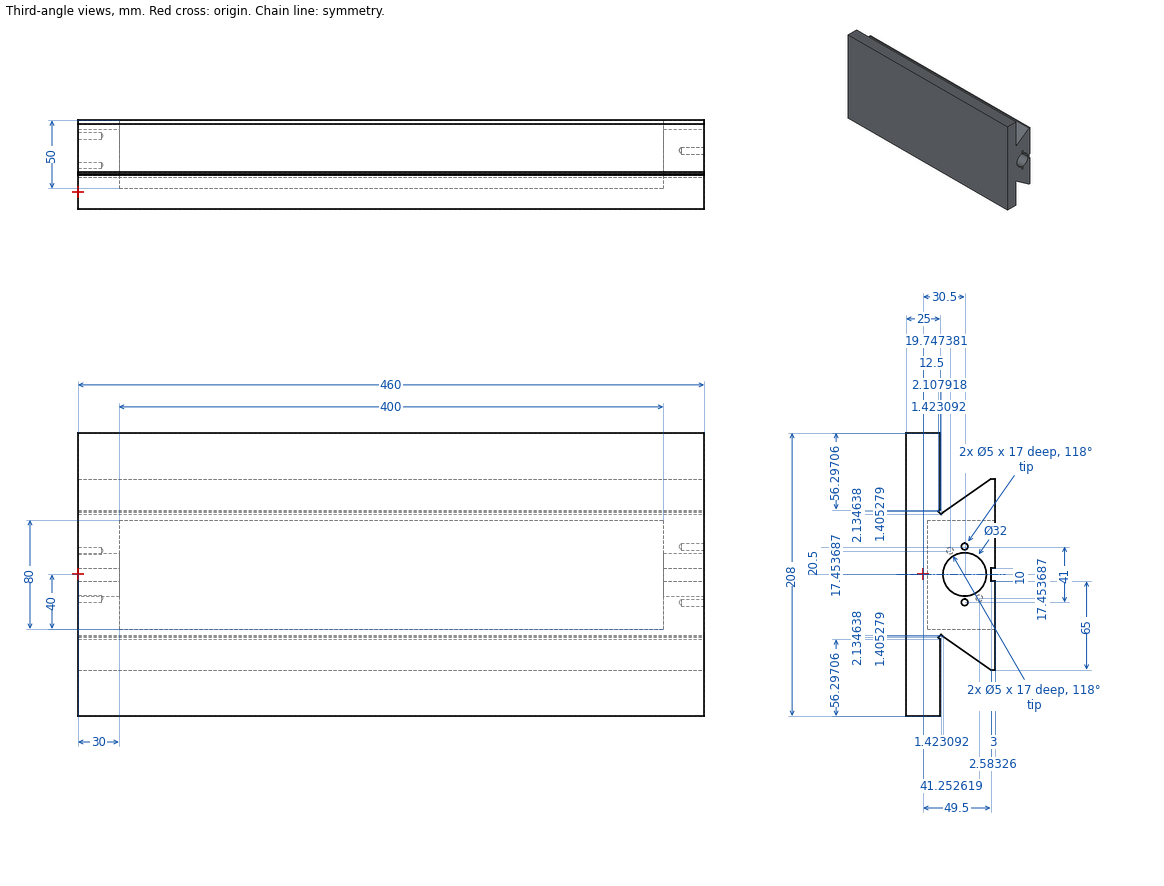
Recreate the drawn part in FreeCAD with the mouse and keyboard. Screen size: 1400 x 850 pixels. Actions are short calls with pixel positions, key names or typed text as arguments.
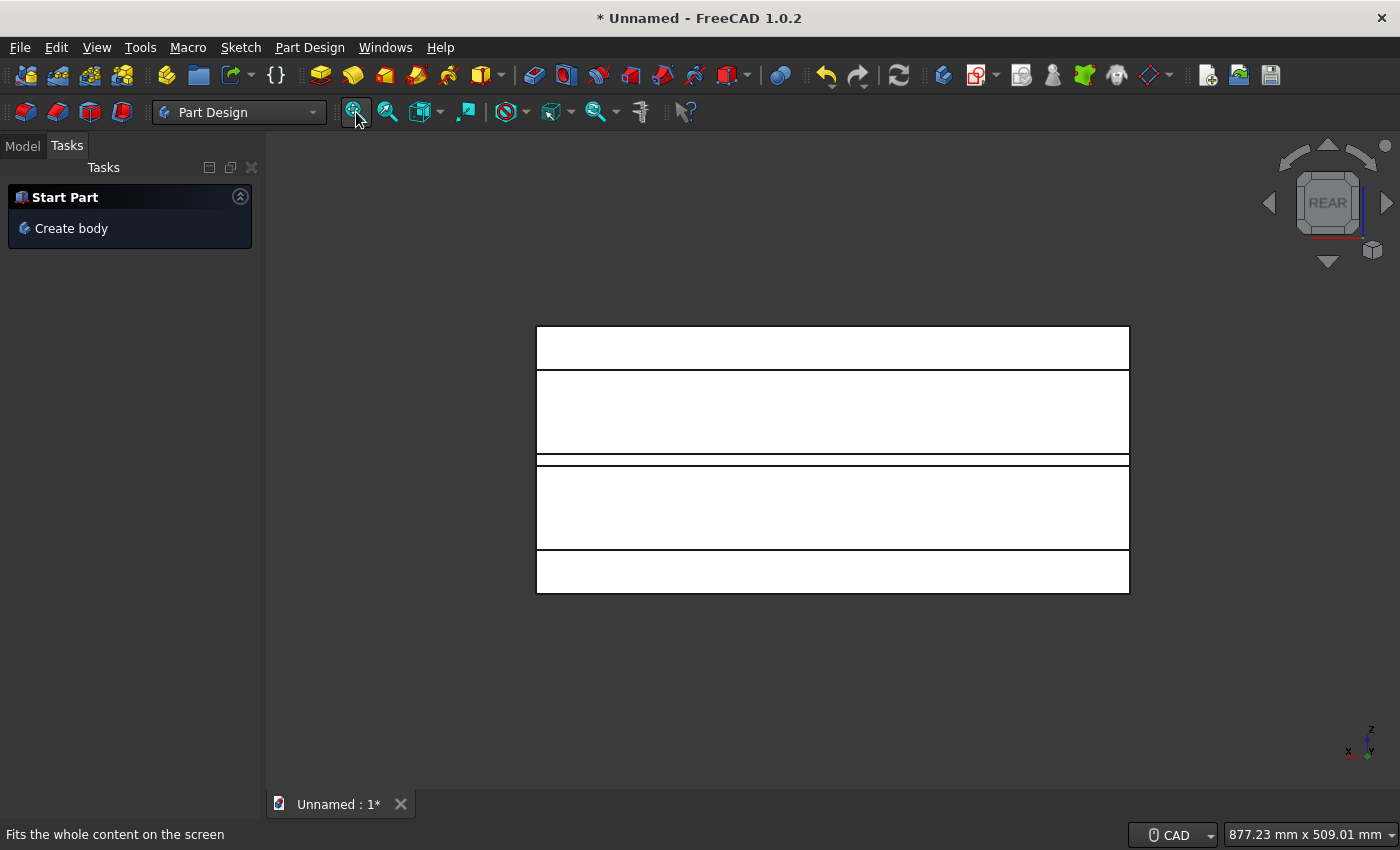
click(833, 411)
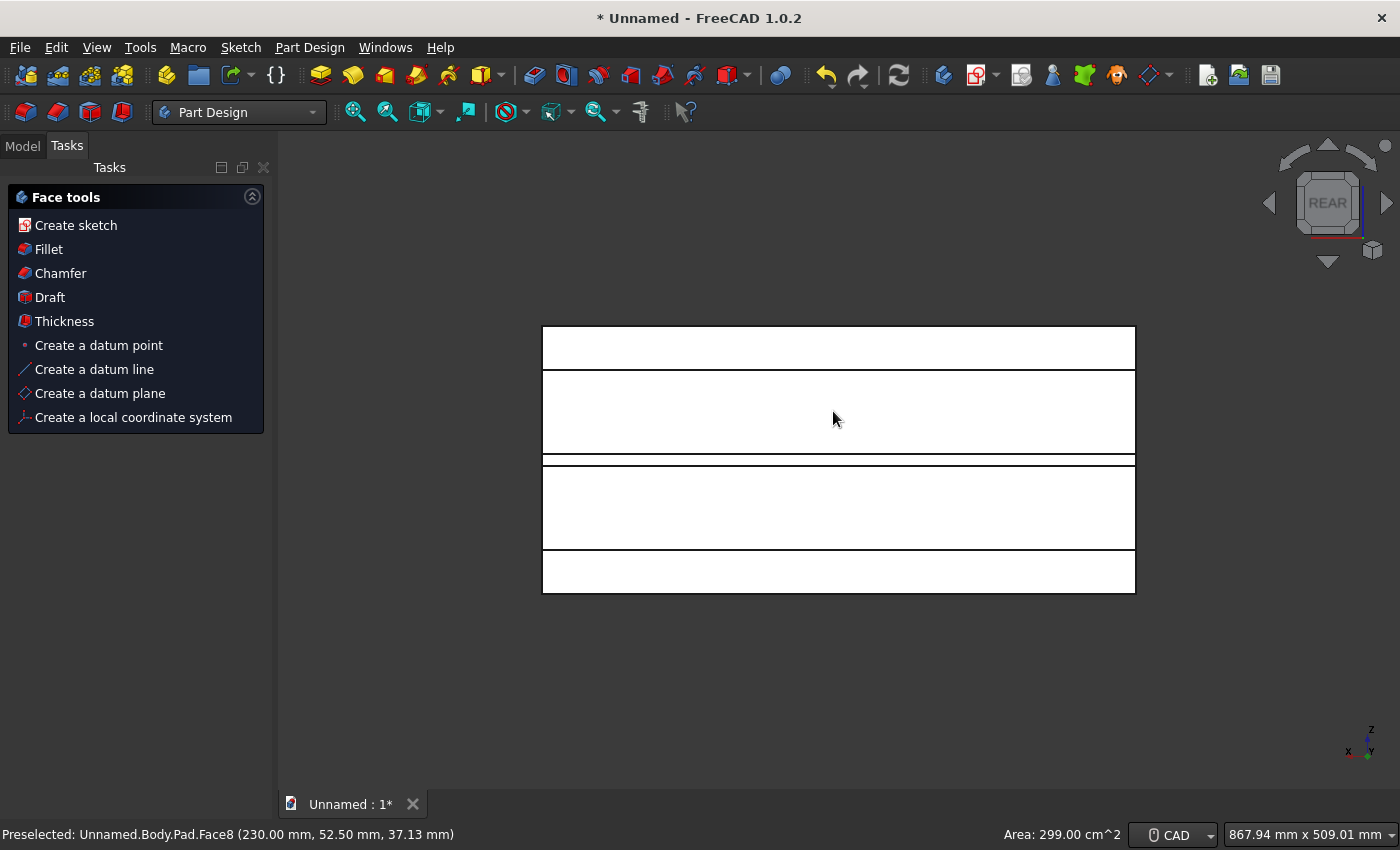
click(976, 76)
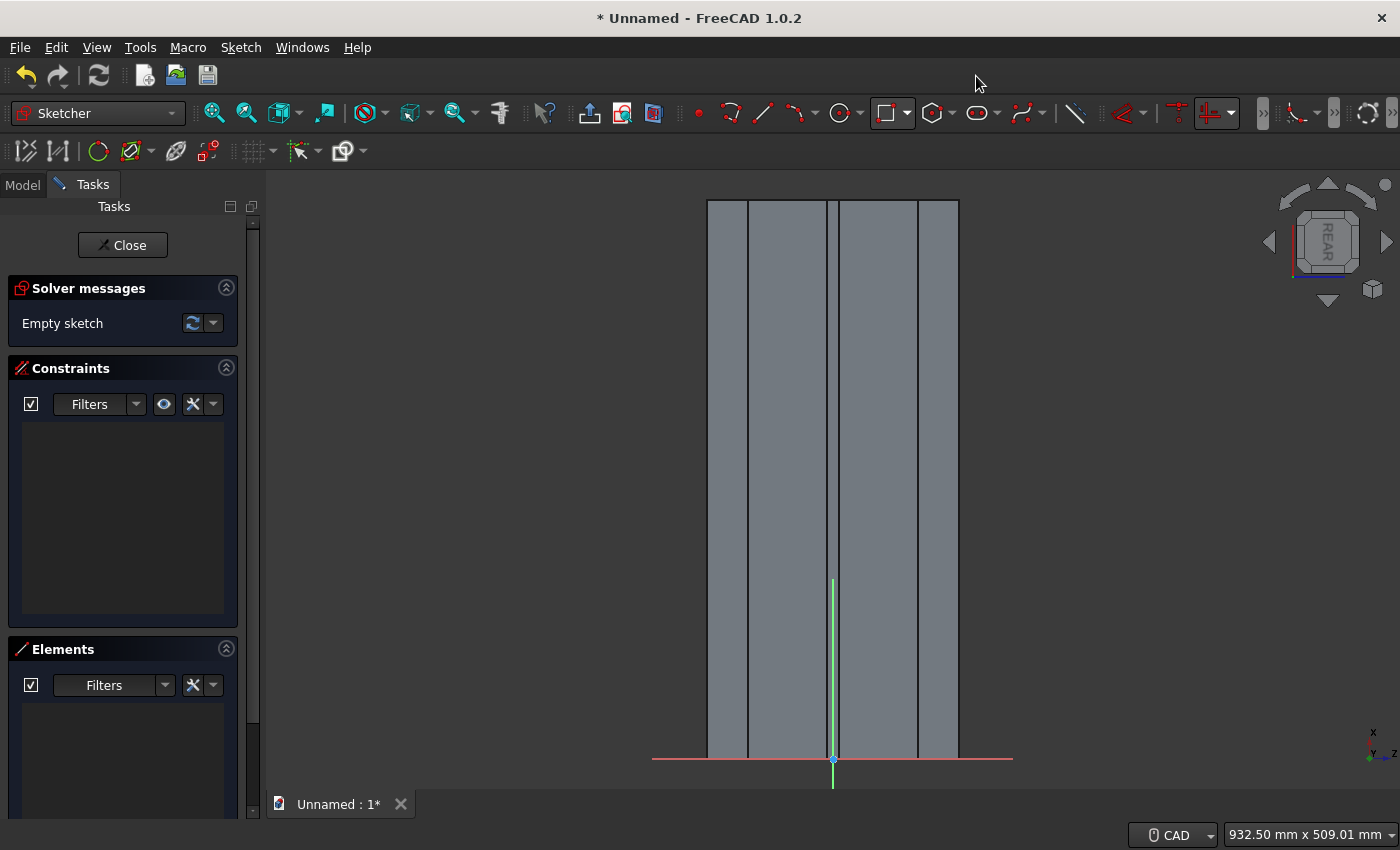
scroll(455, 397, down, 1)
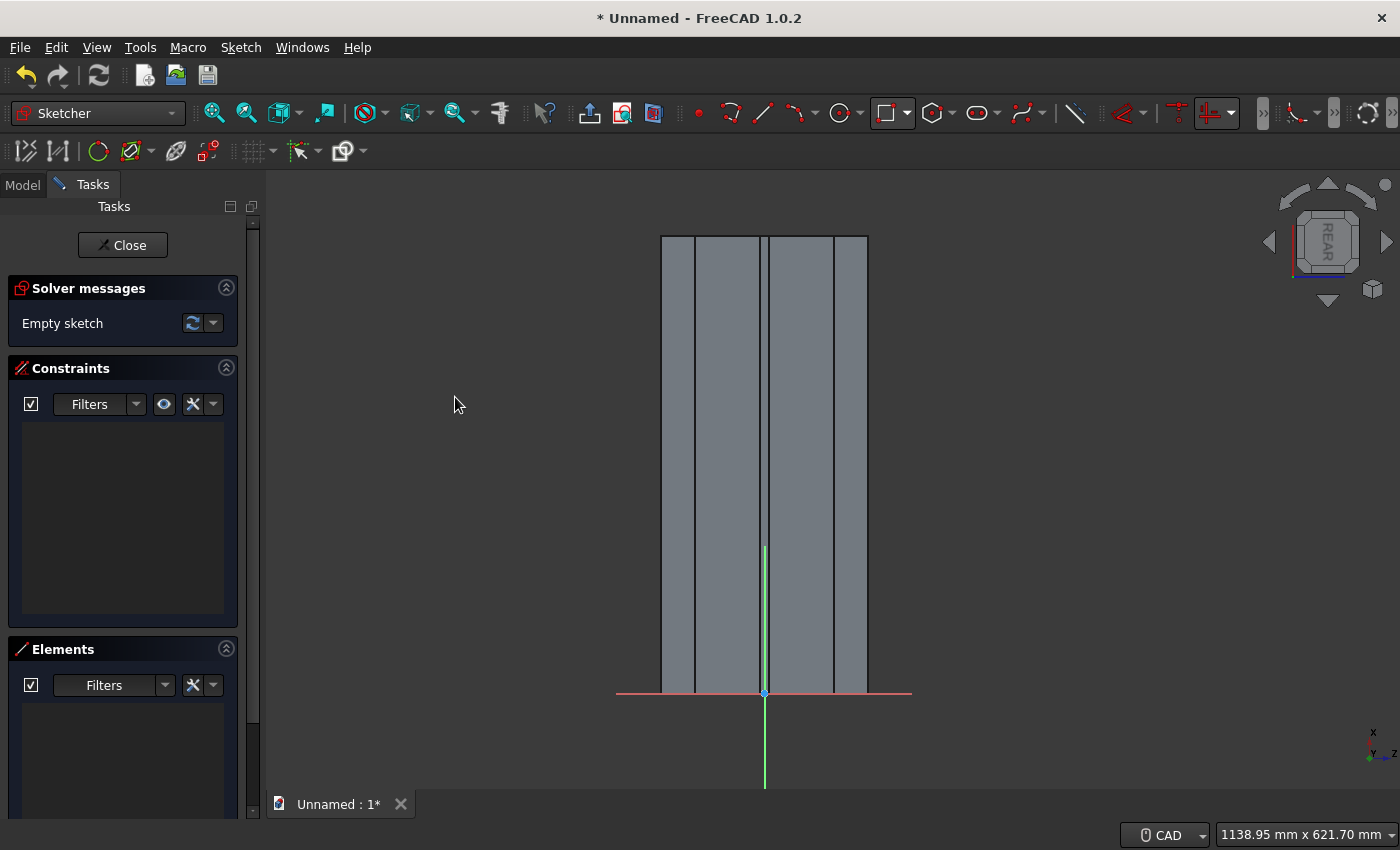
click(886, 114)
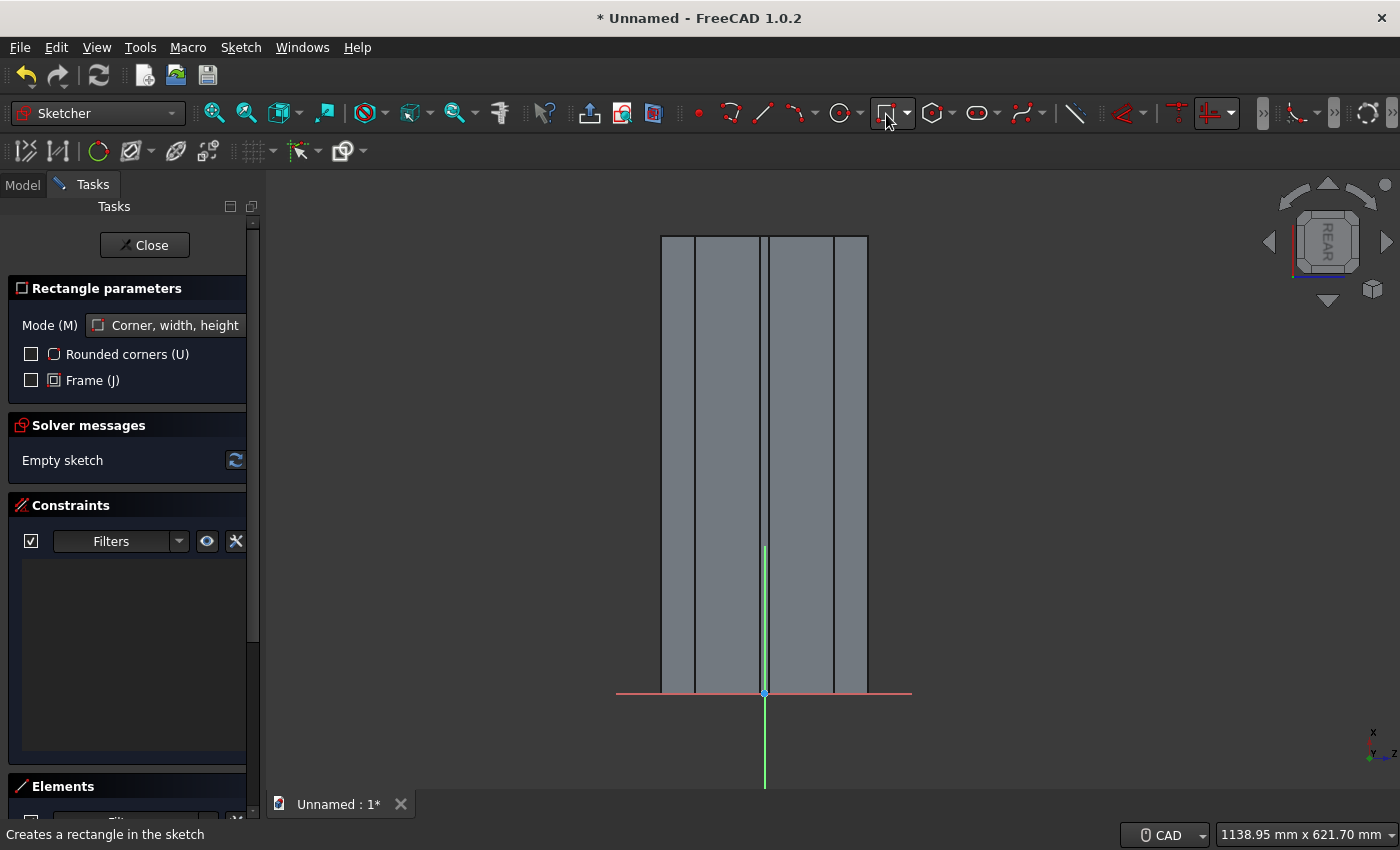
click(725, 265)
move(804, 664)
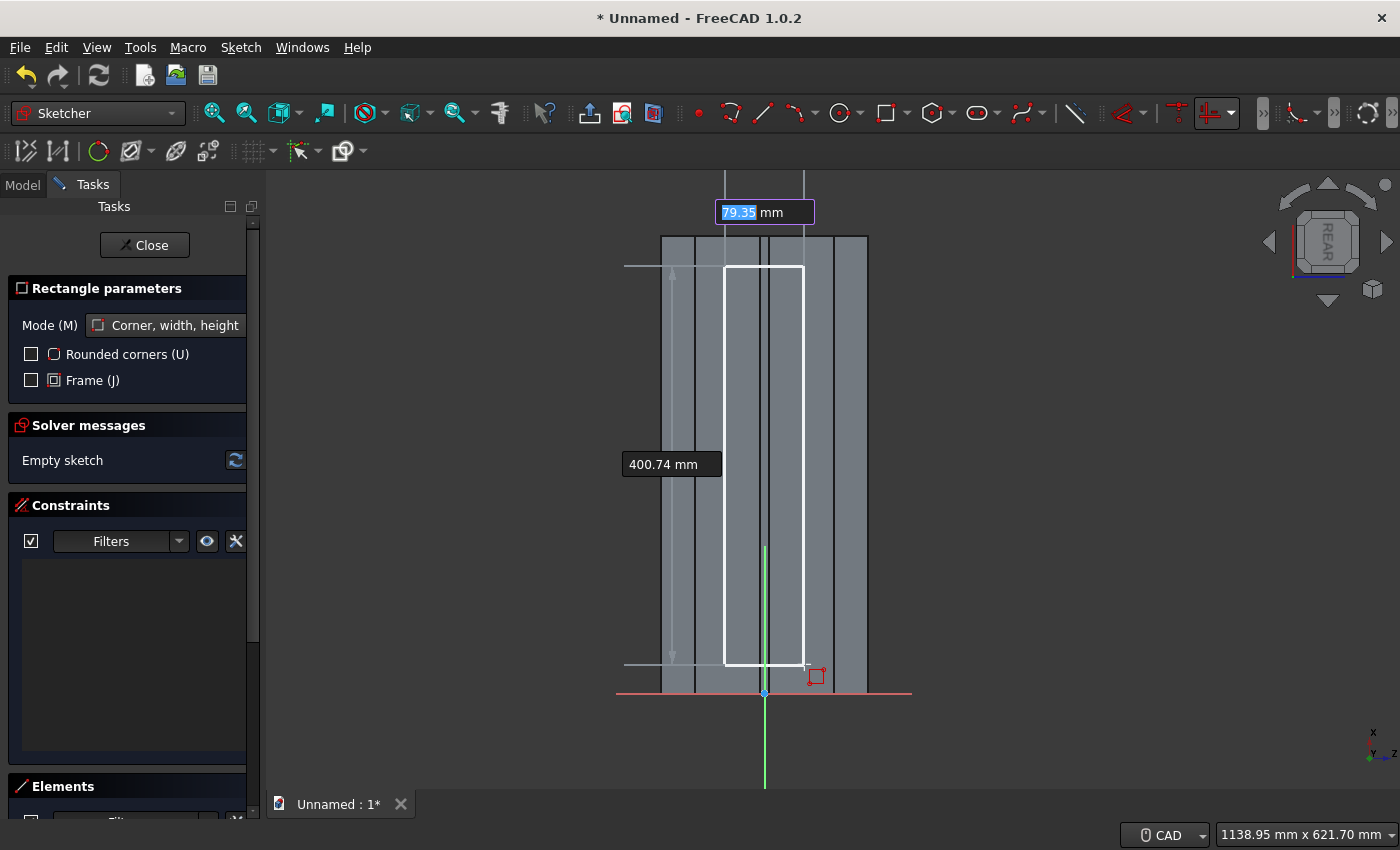
text(80)
key(Tab)
text(400)
key(Return)
key(Escape)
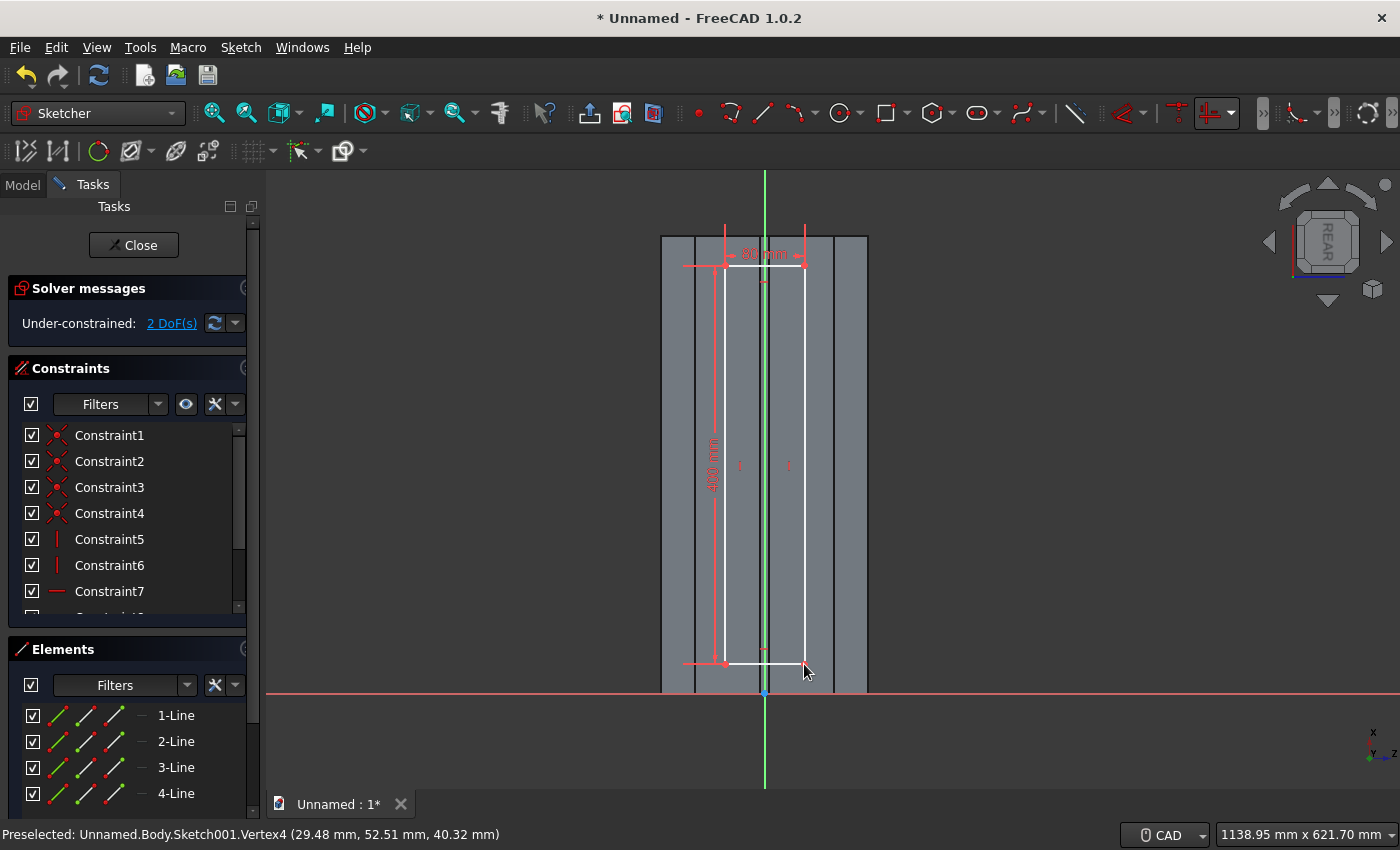
click(1122, 114)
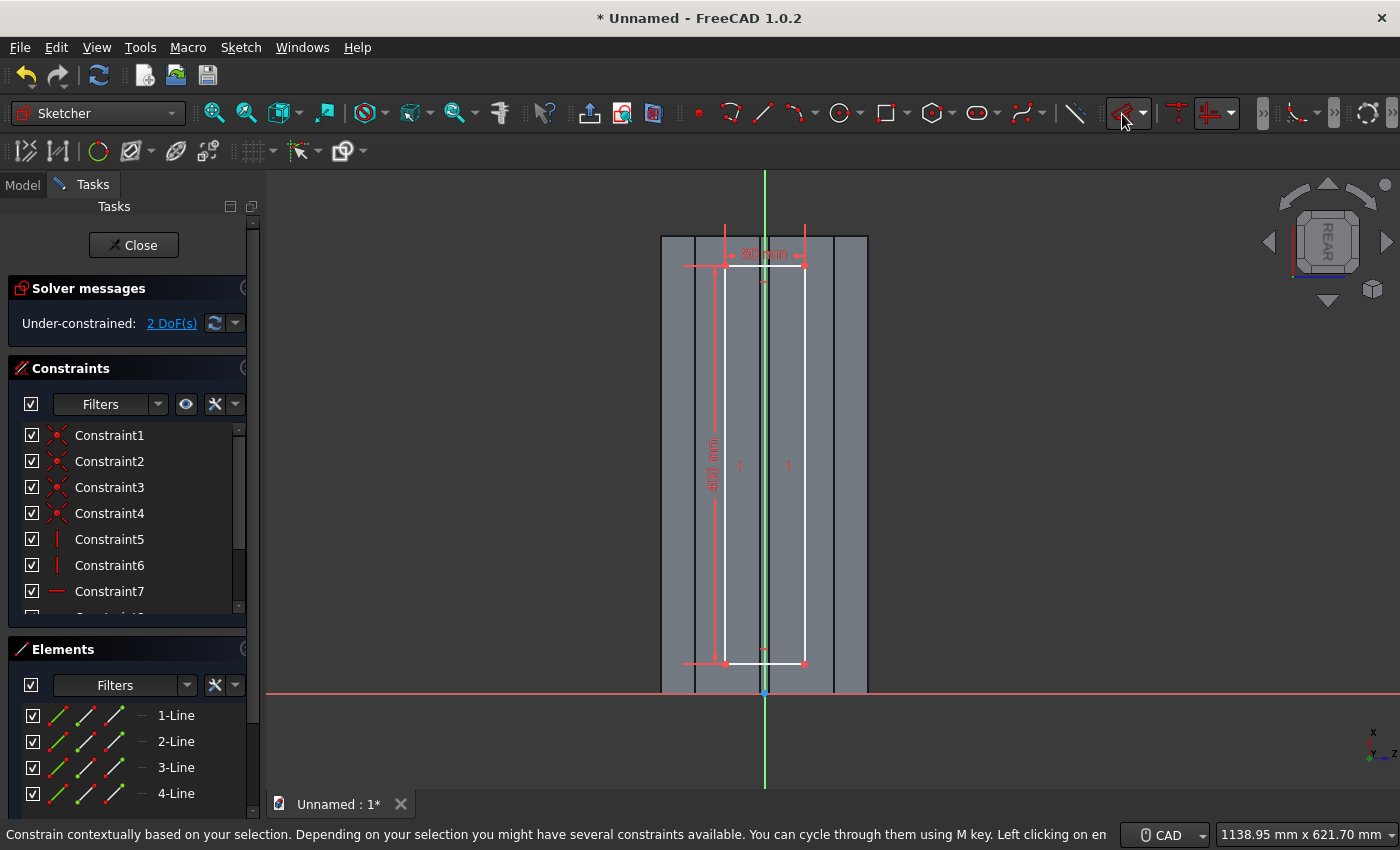
click(725, 266)
click(745, 728)